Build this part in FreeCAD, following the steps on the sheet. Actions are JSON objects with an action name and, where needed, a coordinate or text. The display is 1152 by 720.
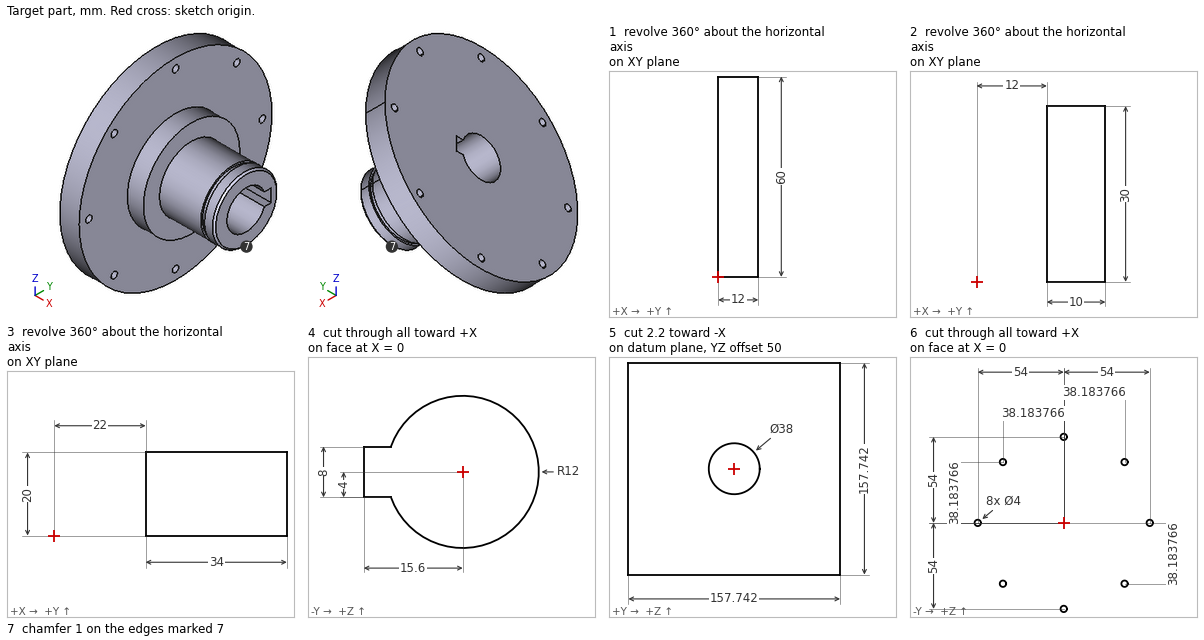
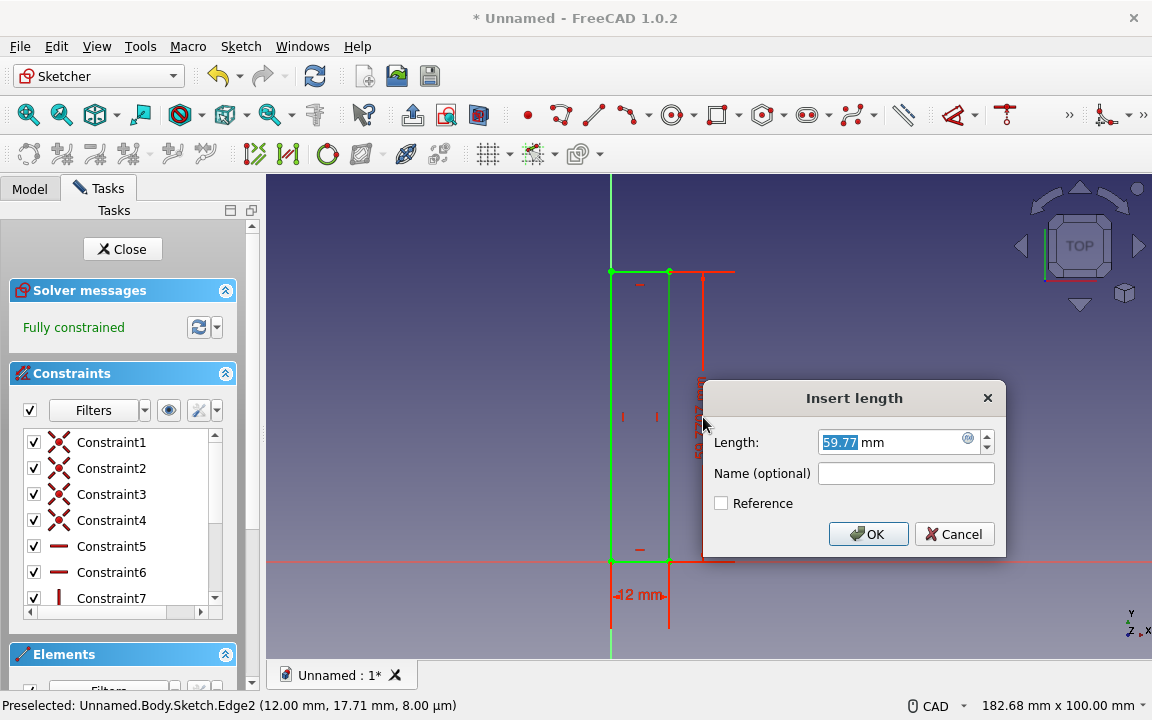
{"action": "type", "text": "60"}
{"action": "key", "text": "Return"}
{"action": "key", "text": "Escape"}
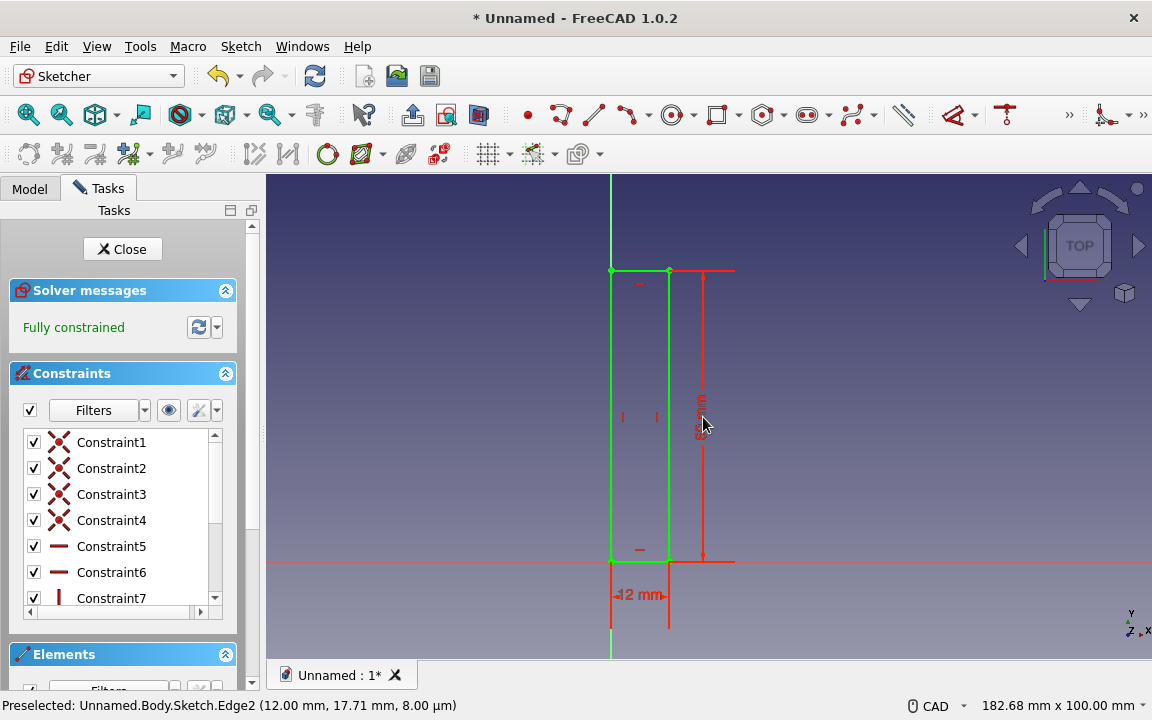
{"action": "left_click", "coordinate": [123, 249]}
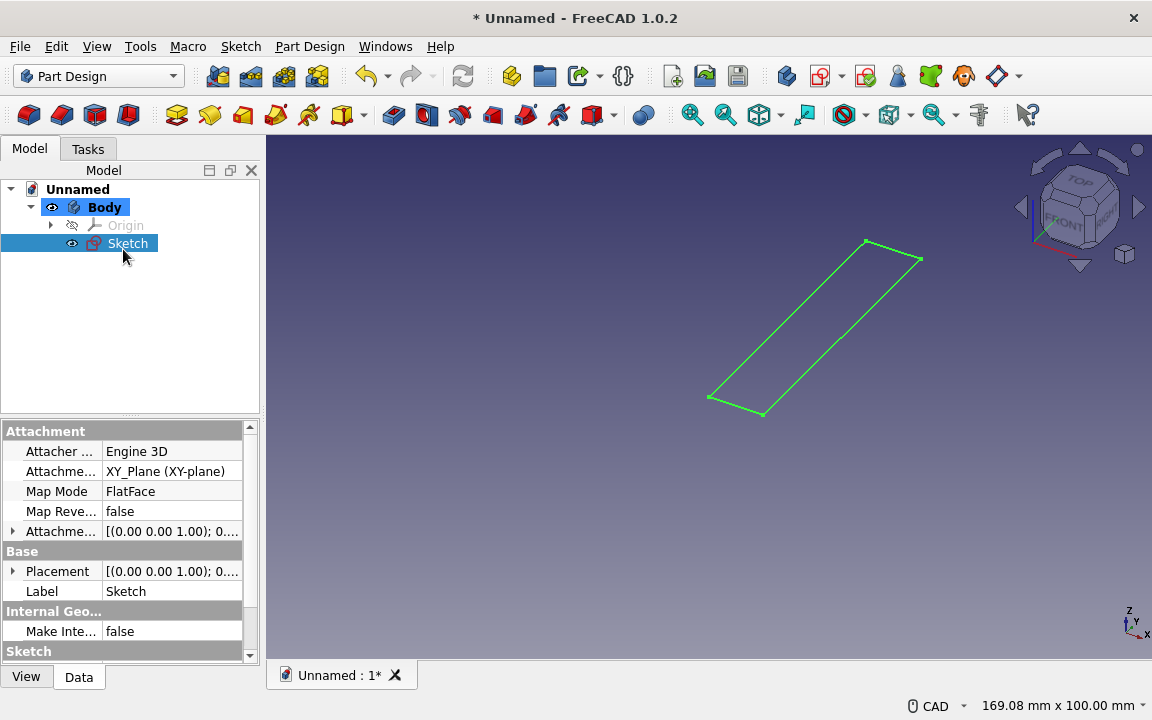
{"action": "left_click", "coordinate": [210, 116]}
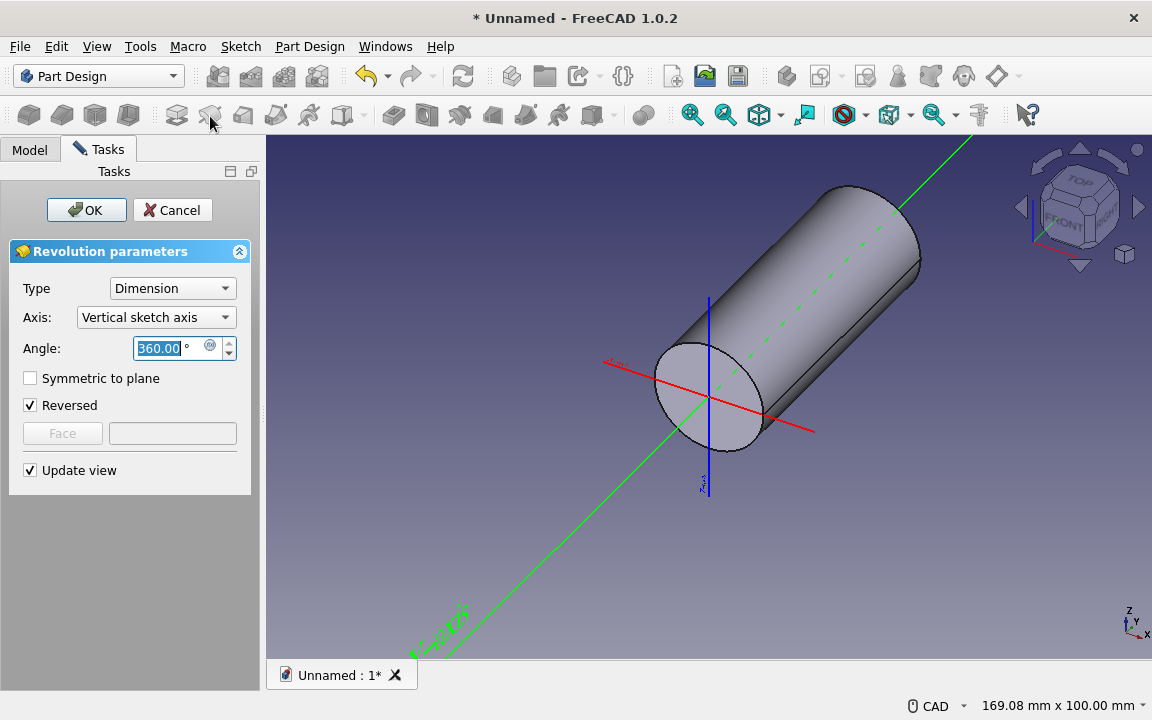
{"action": "left_click", "coordinate": [157, 318]}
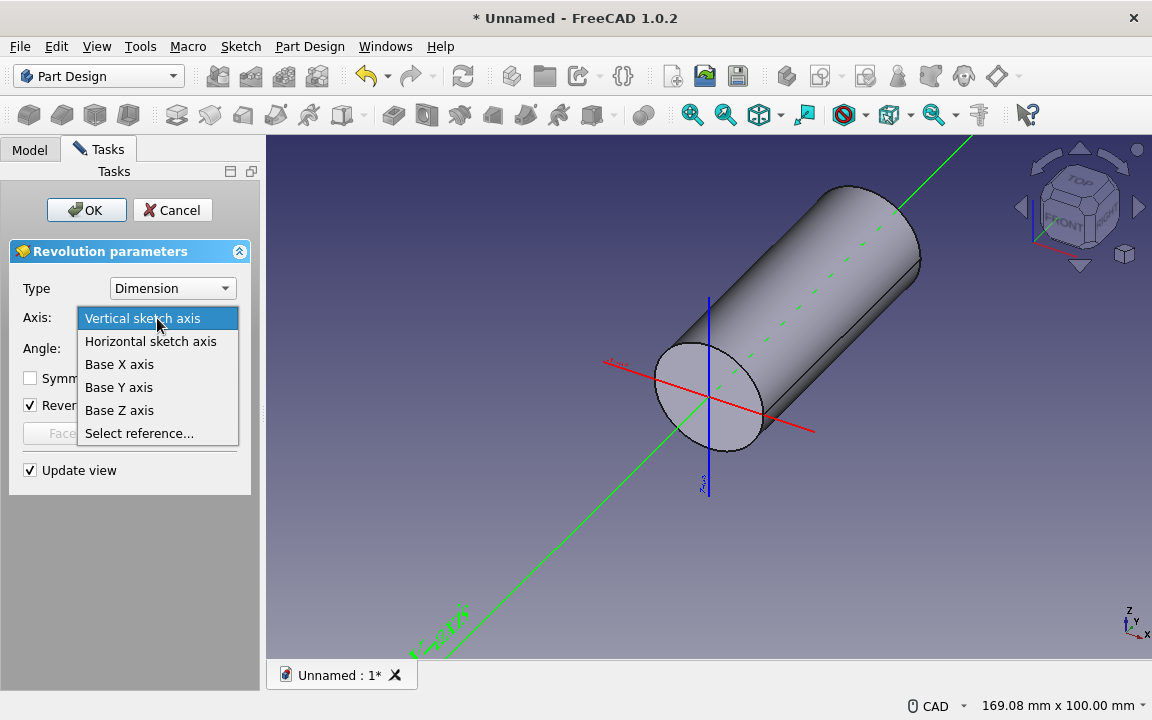
{"action": "left_click", "coordinate": [156, 342]}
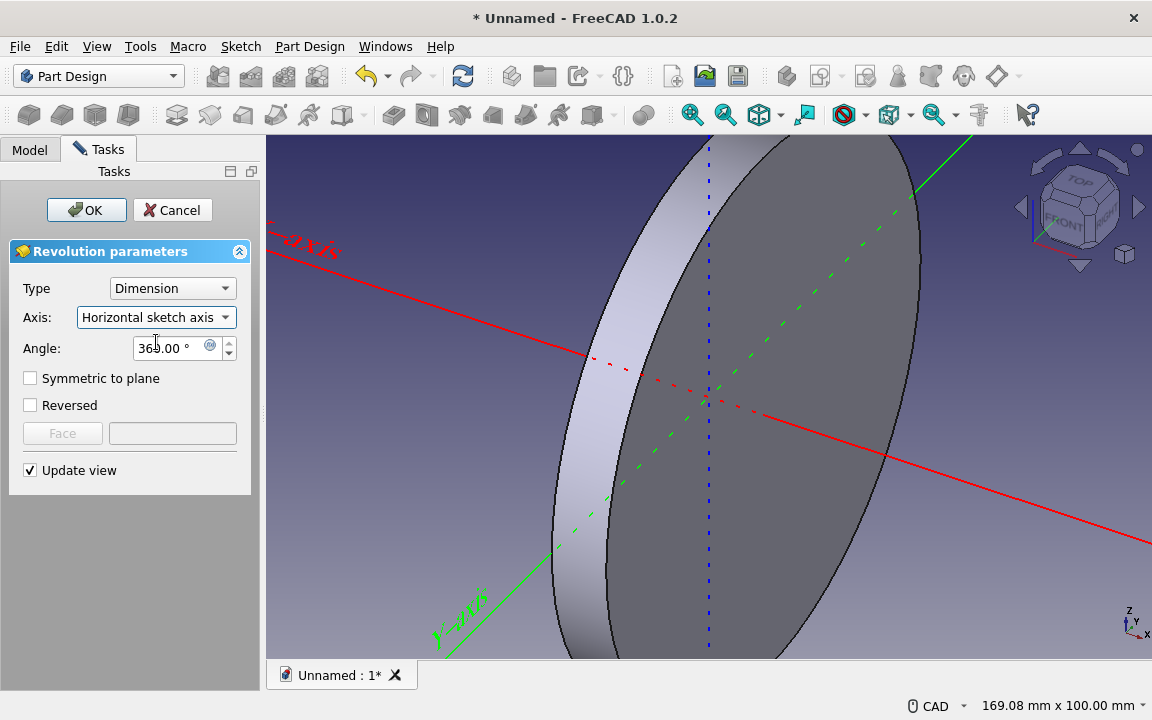
{"action": "left_click", "coordinate": [87, 210]}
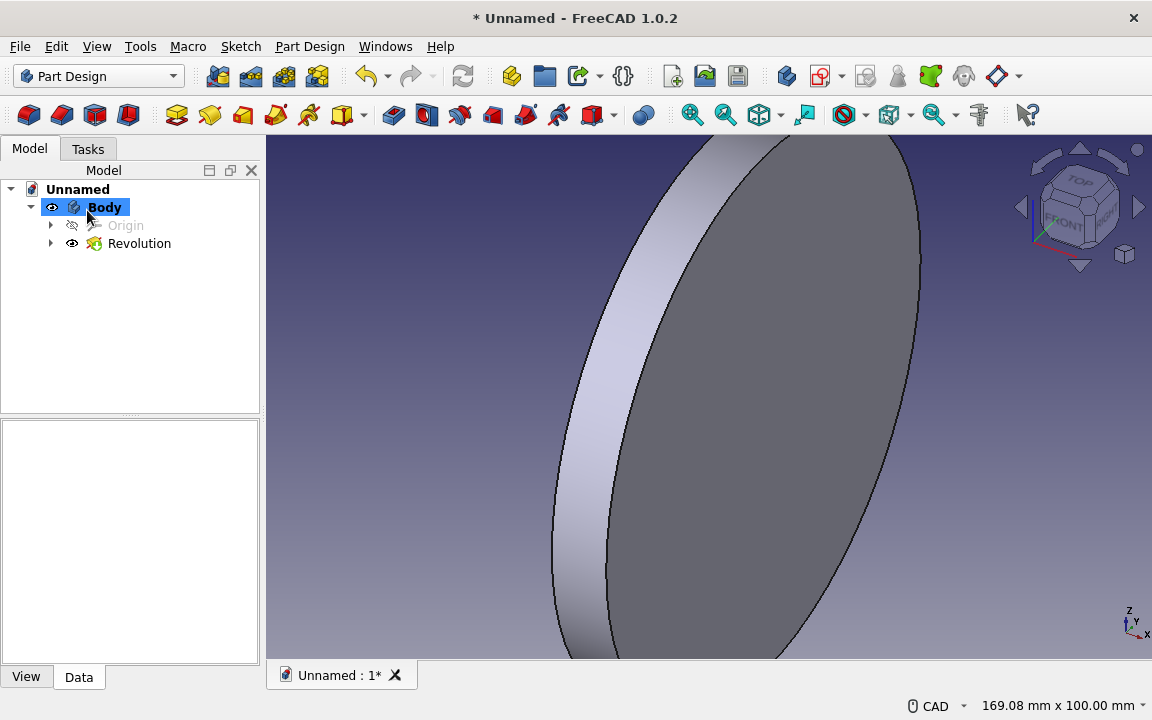
{"action": "left_click", "coordinate": [693, 116]}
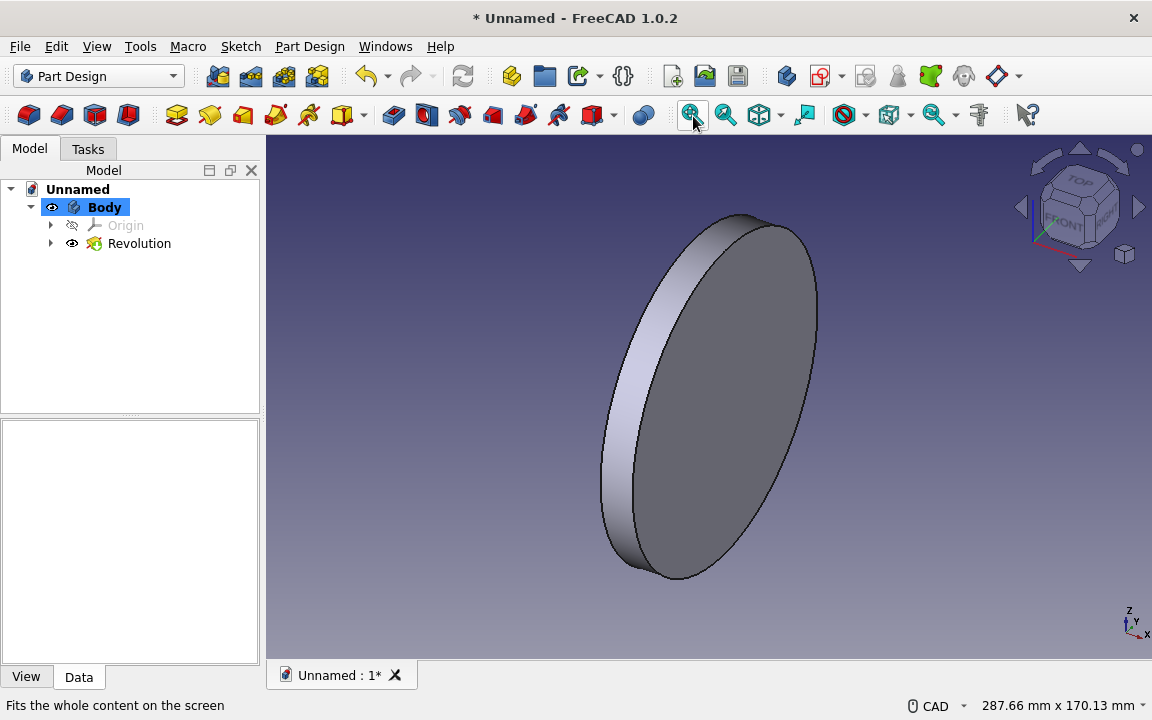
{"action": "left_click", "coordinate": [820, 76]}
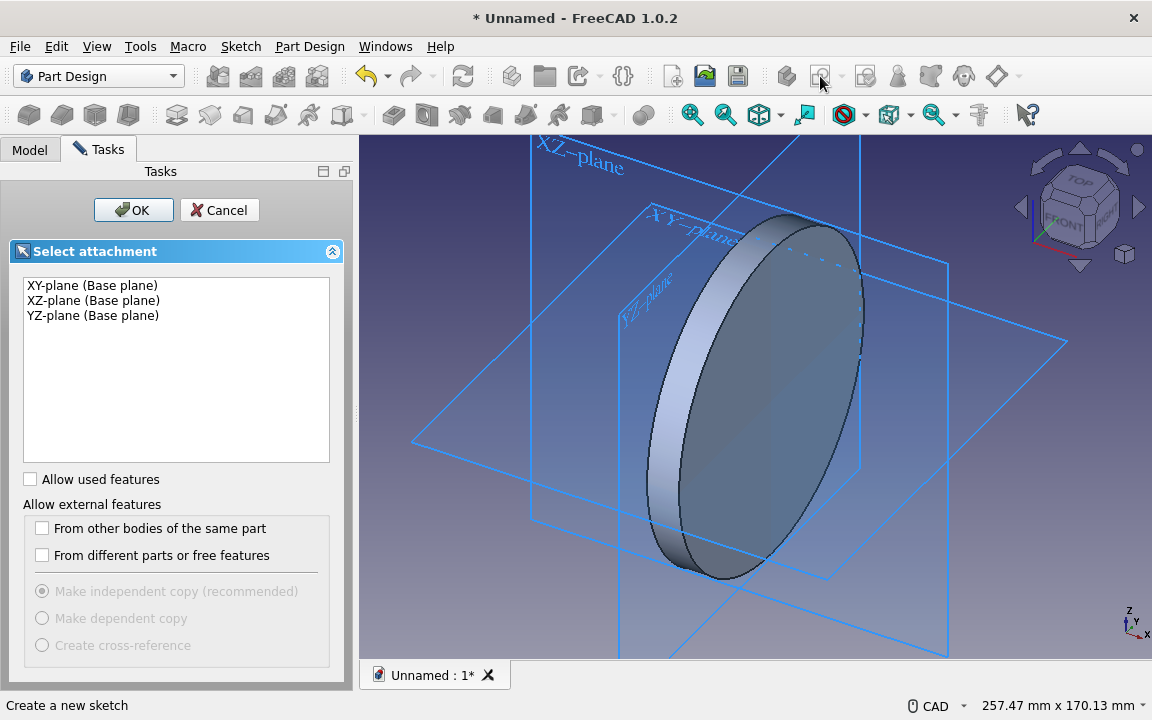
{"action": "left_click", "coordinate": [84, 286]}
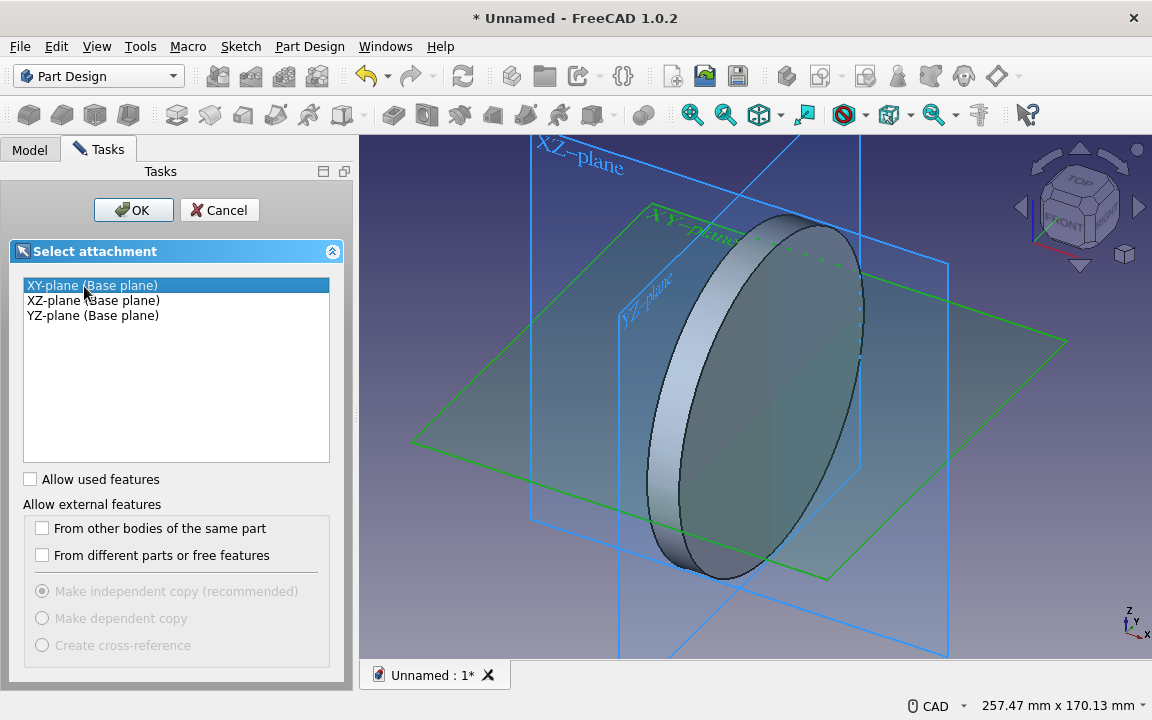
{"action": "left_click", "coordinate": [134, 210]}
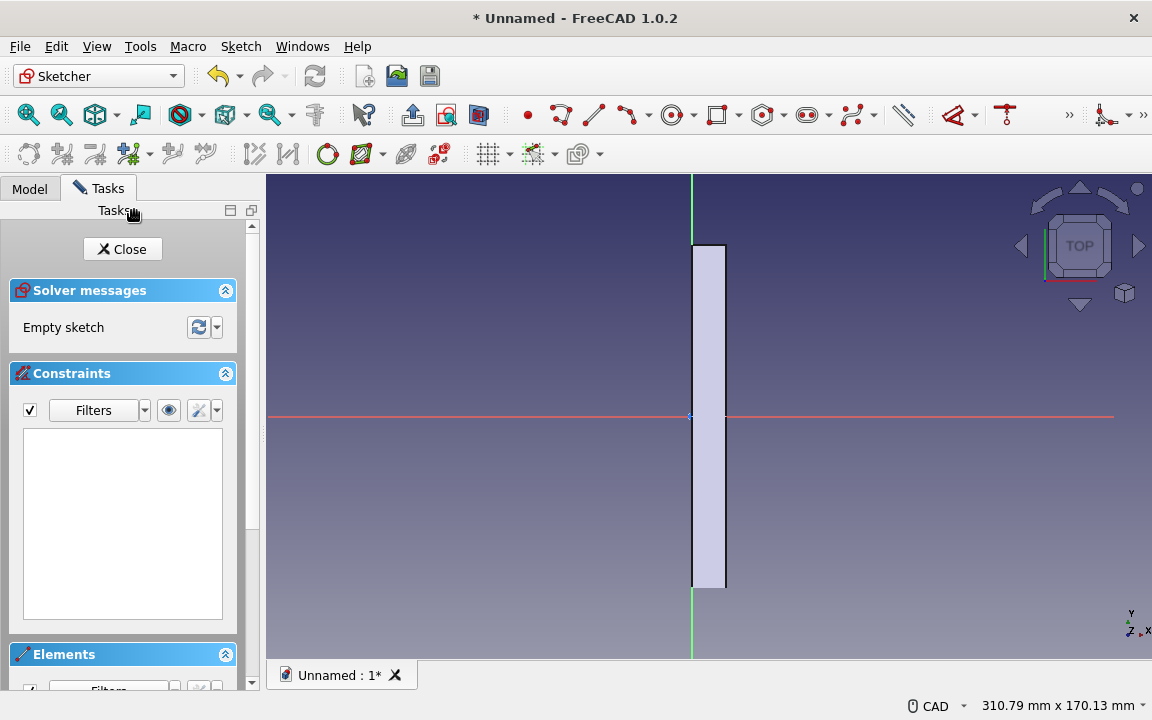
{"action": "left_click", "coordinate": [479, 116]}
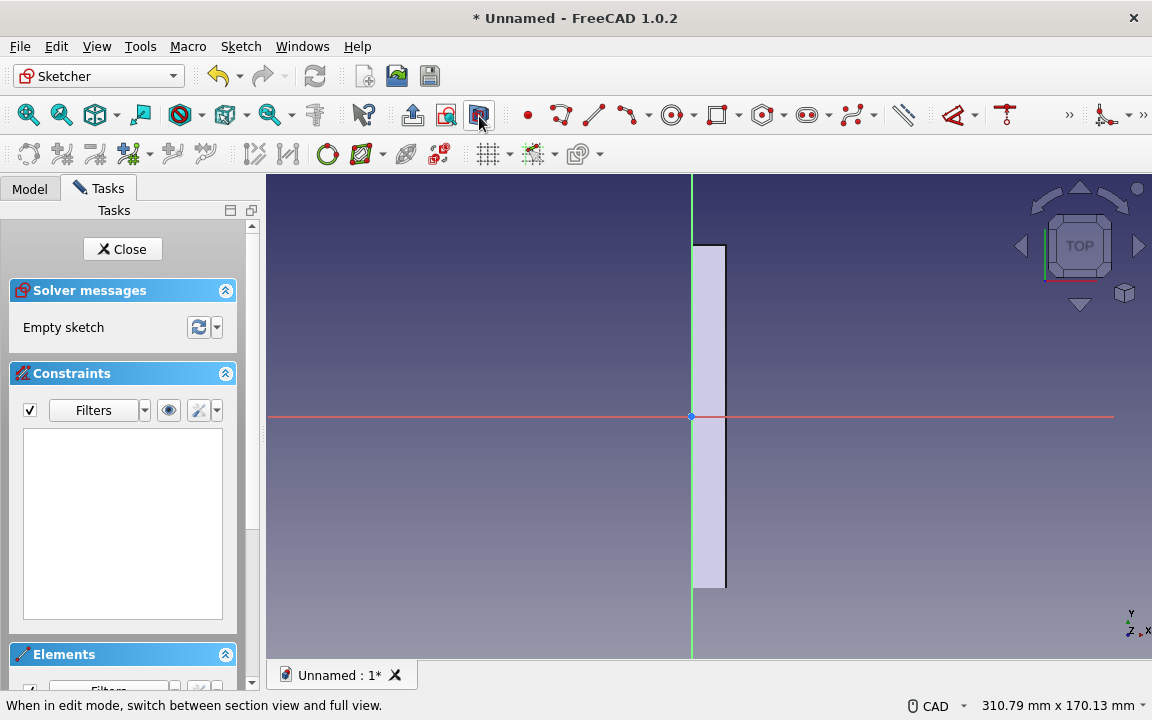
{"action": "scroll", "coordinate": [759, 355], "scroll_direction": "up", "scroll_amount": 6}